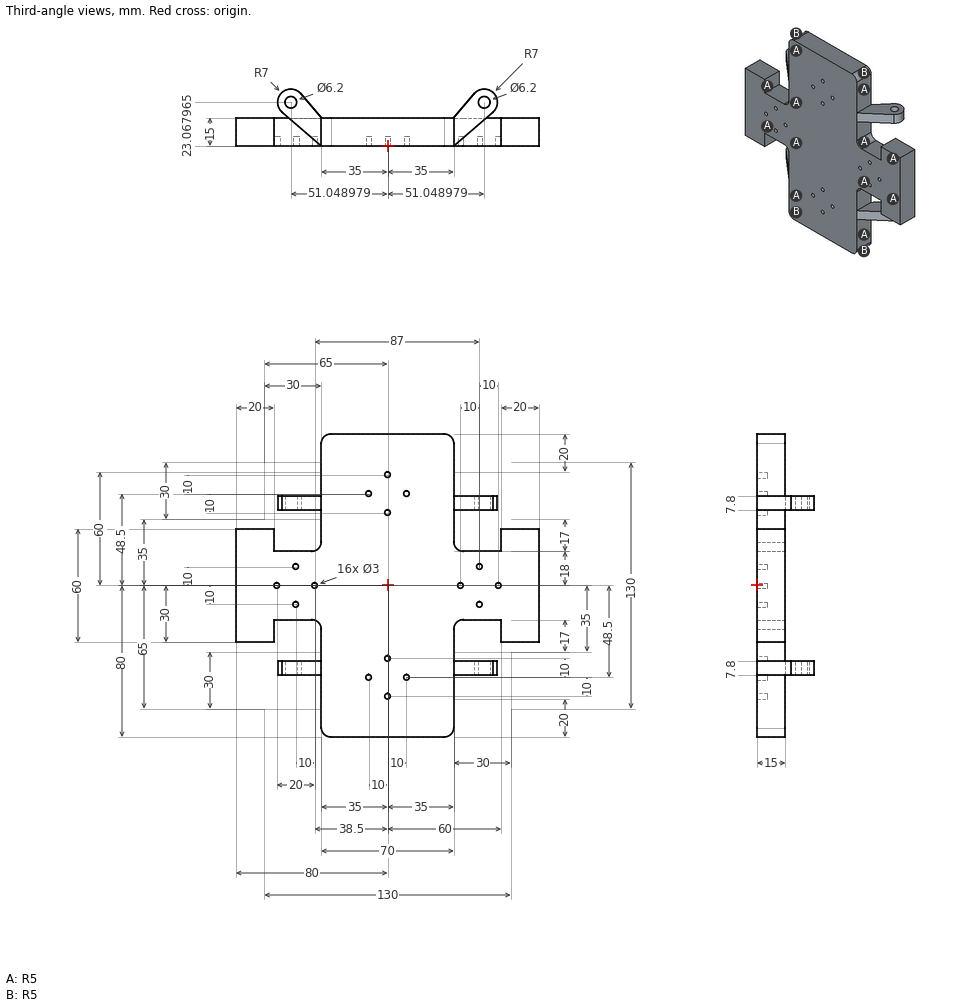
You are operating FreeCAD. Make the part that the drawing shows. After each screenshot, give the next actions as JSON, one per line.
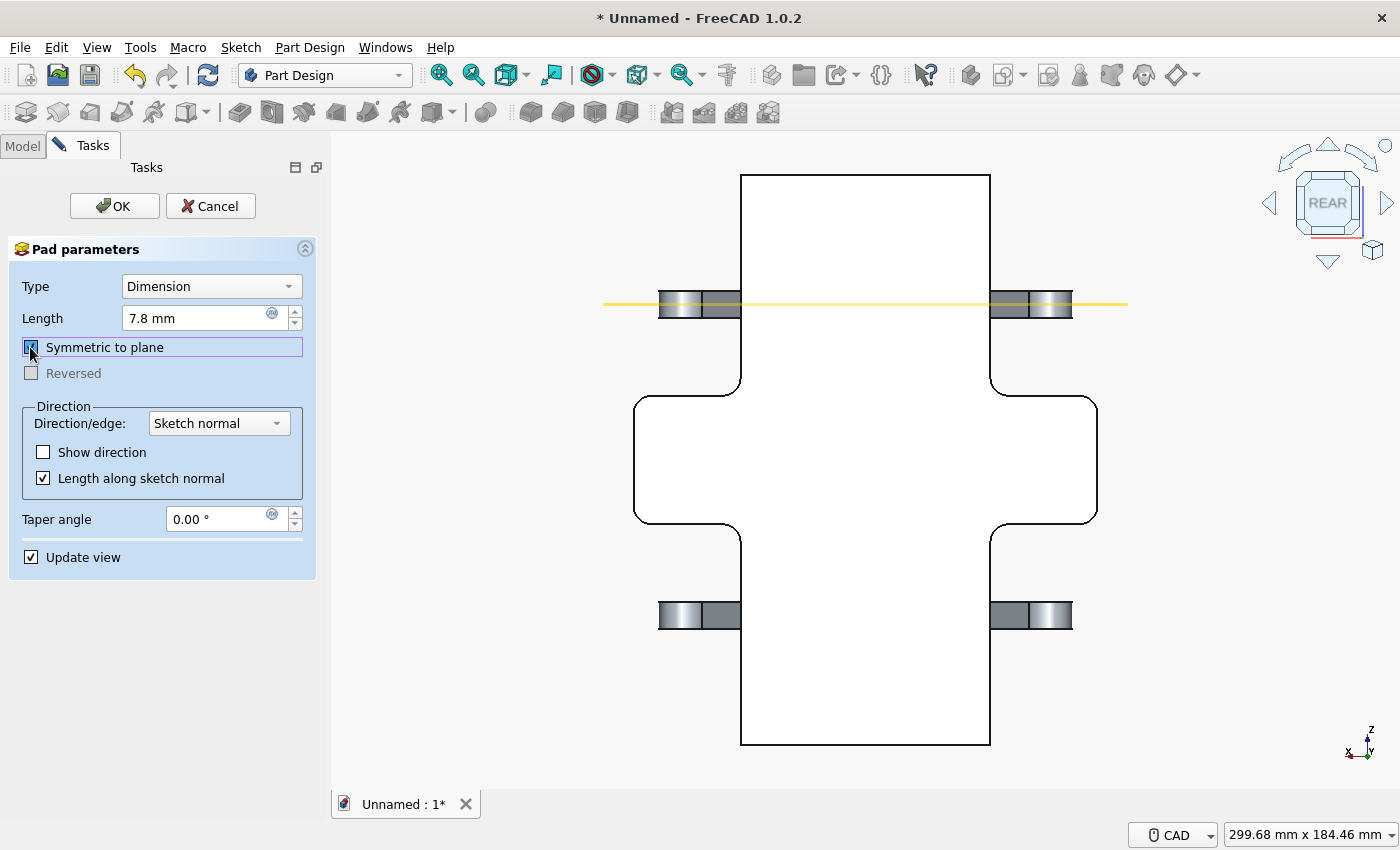
{"action": "left_click", "coordinate": [115, 206]}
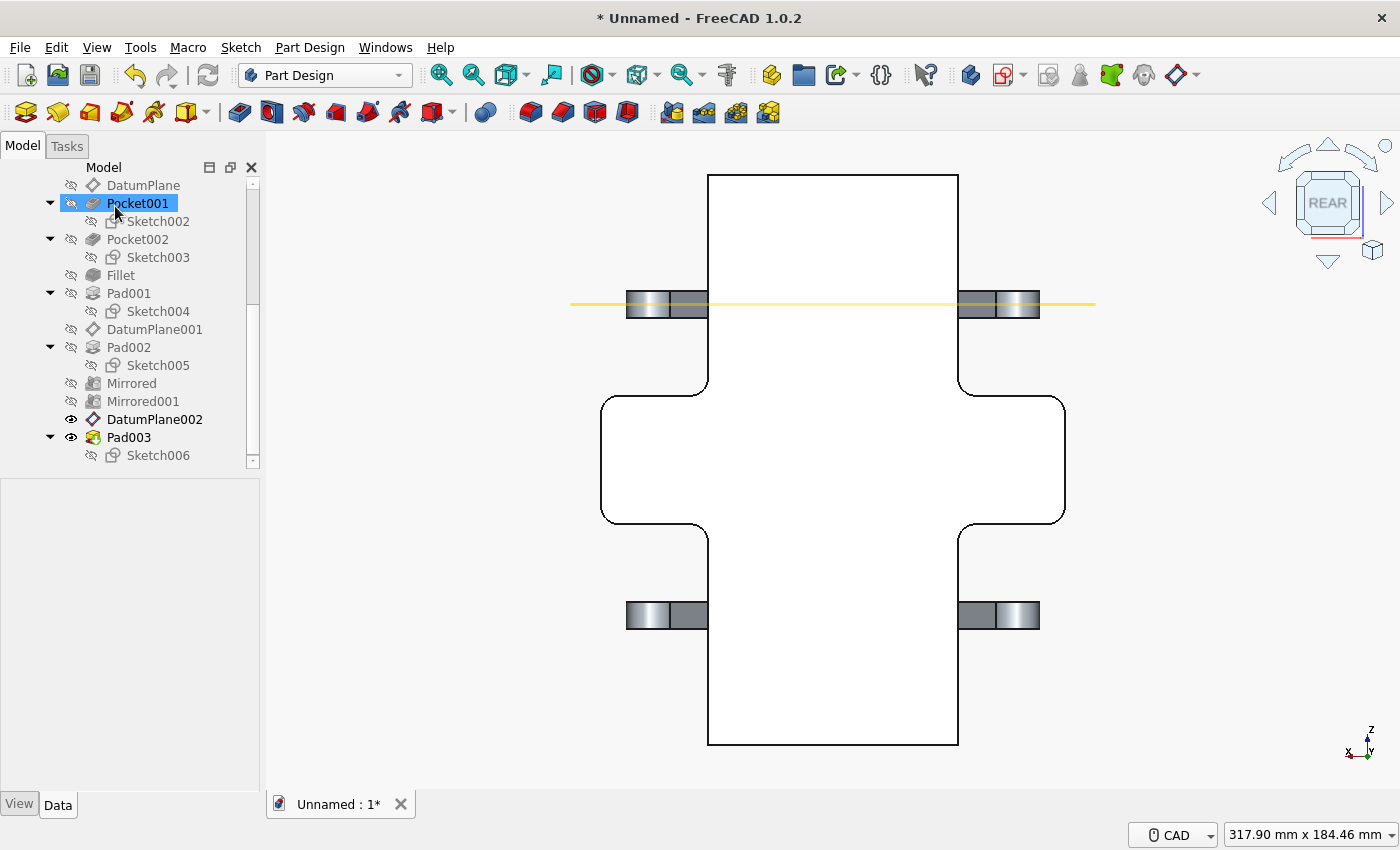
{"action": "left_click", "coordinate": [116, 419]}
{"action": "key", "text": "space"}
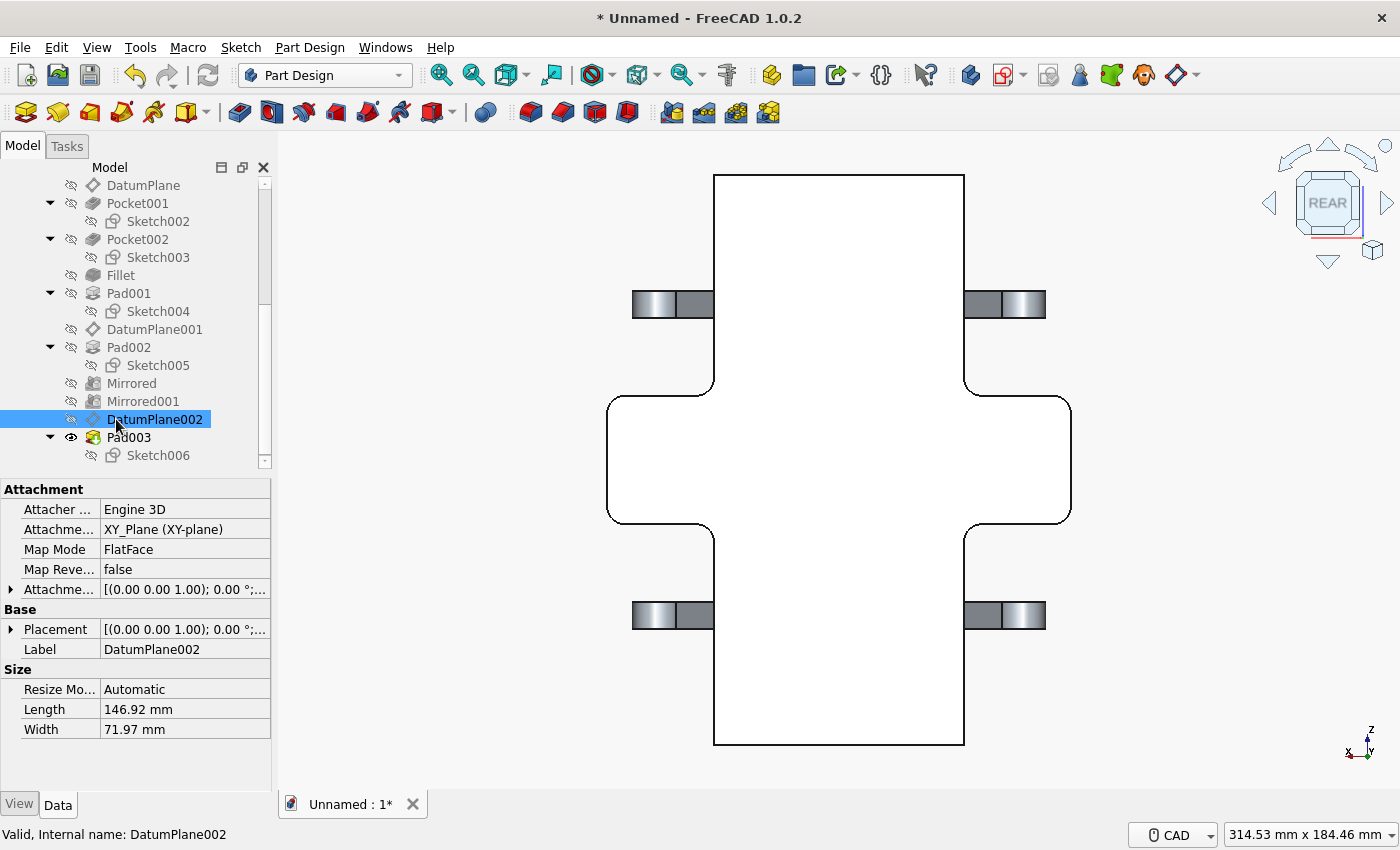
{"action": "key", "text": "0"}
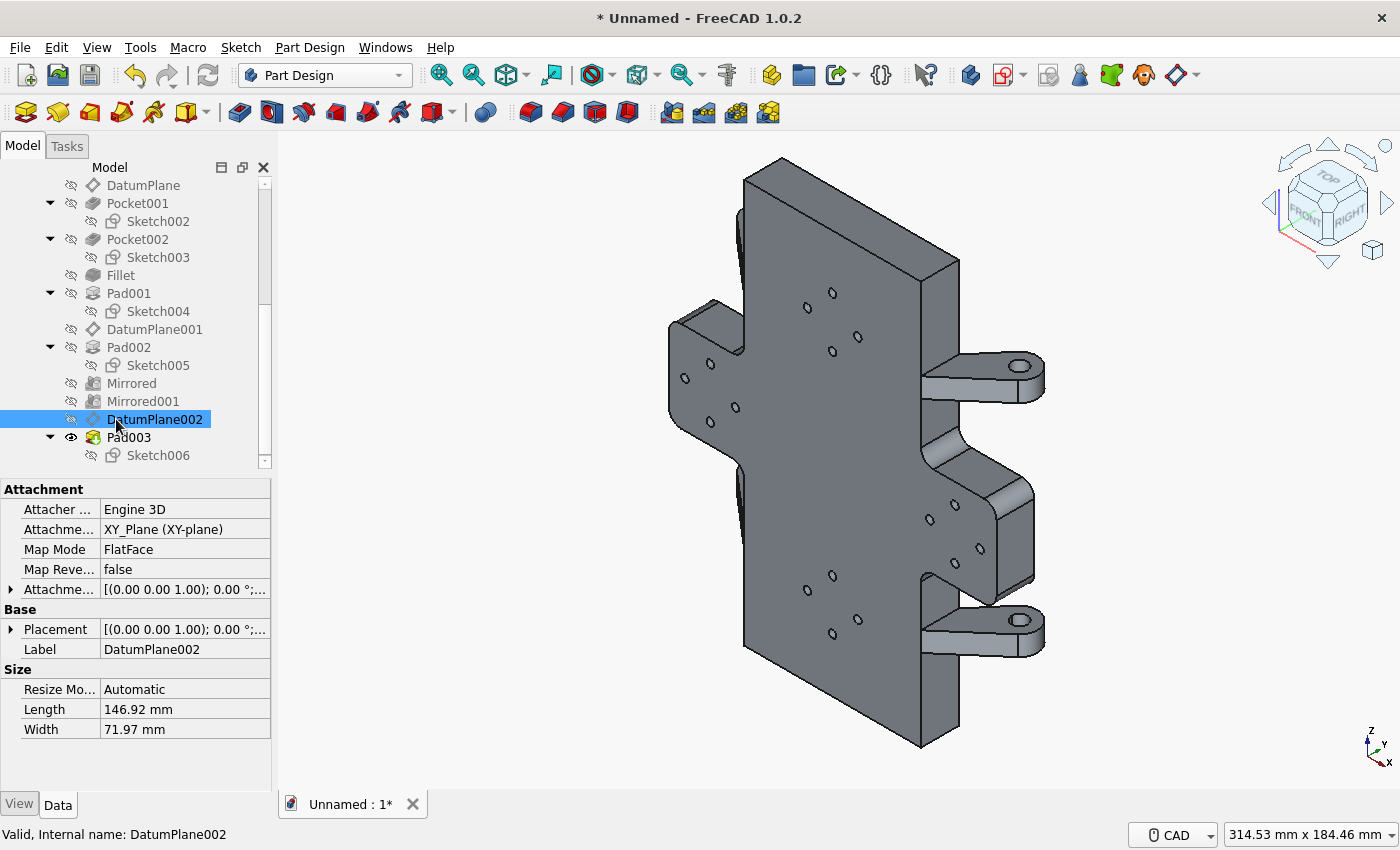
{"action": "key", "text": "v f"}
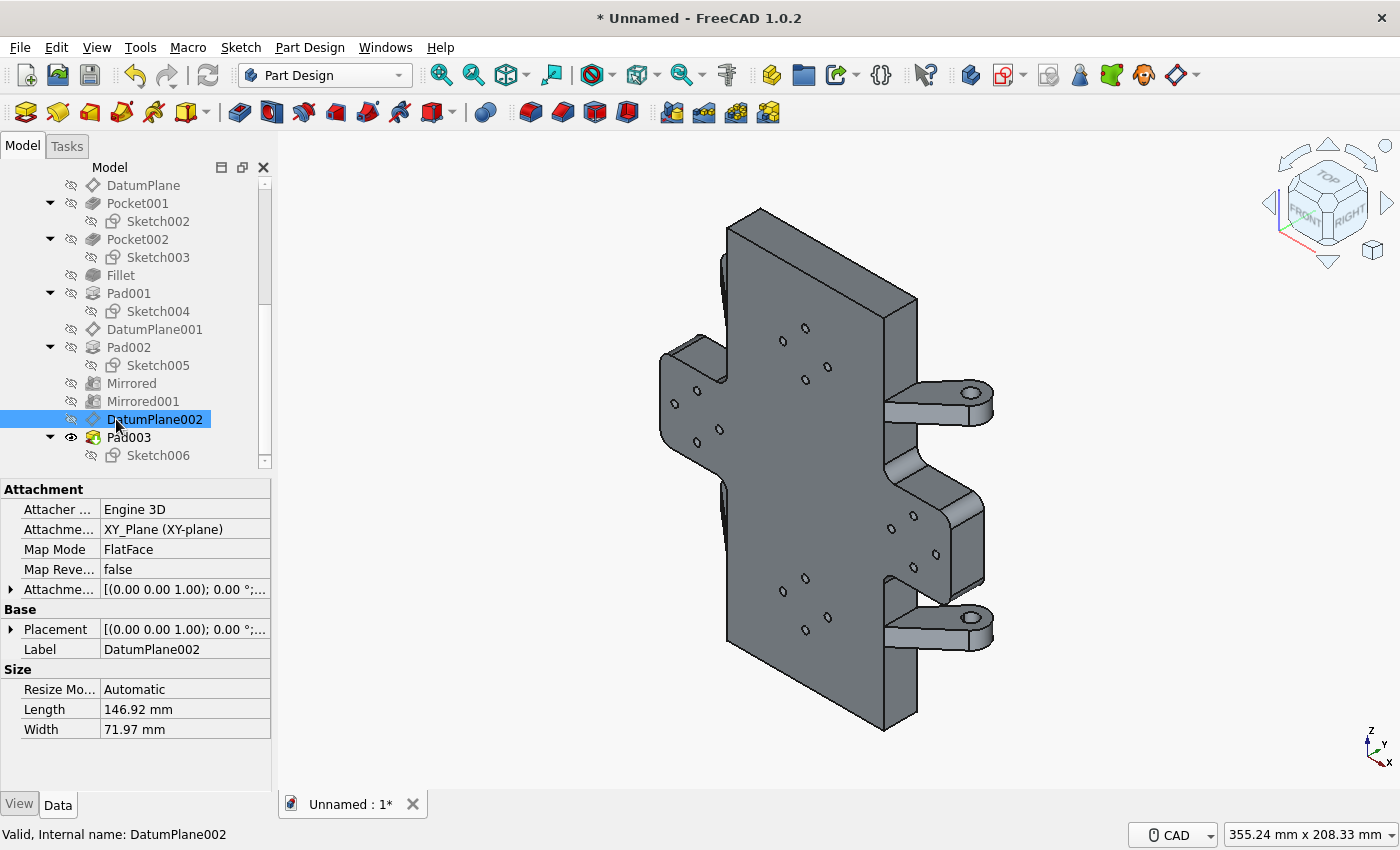
{"action": "left_click", "coordinate": [900, 308]}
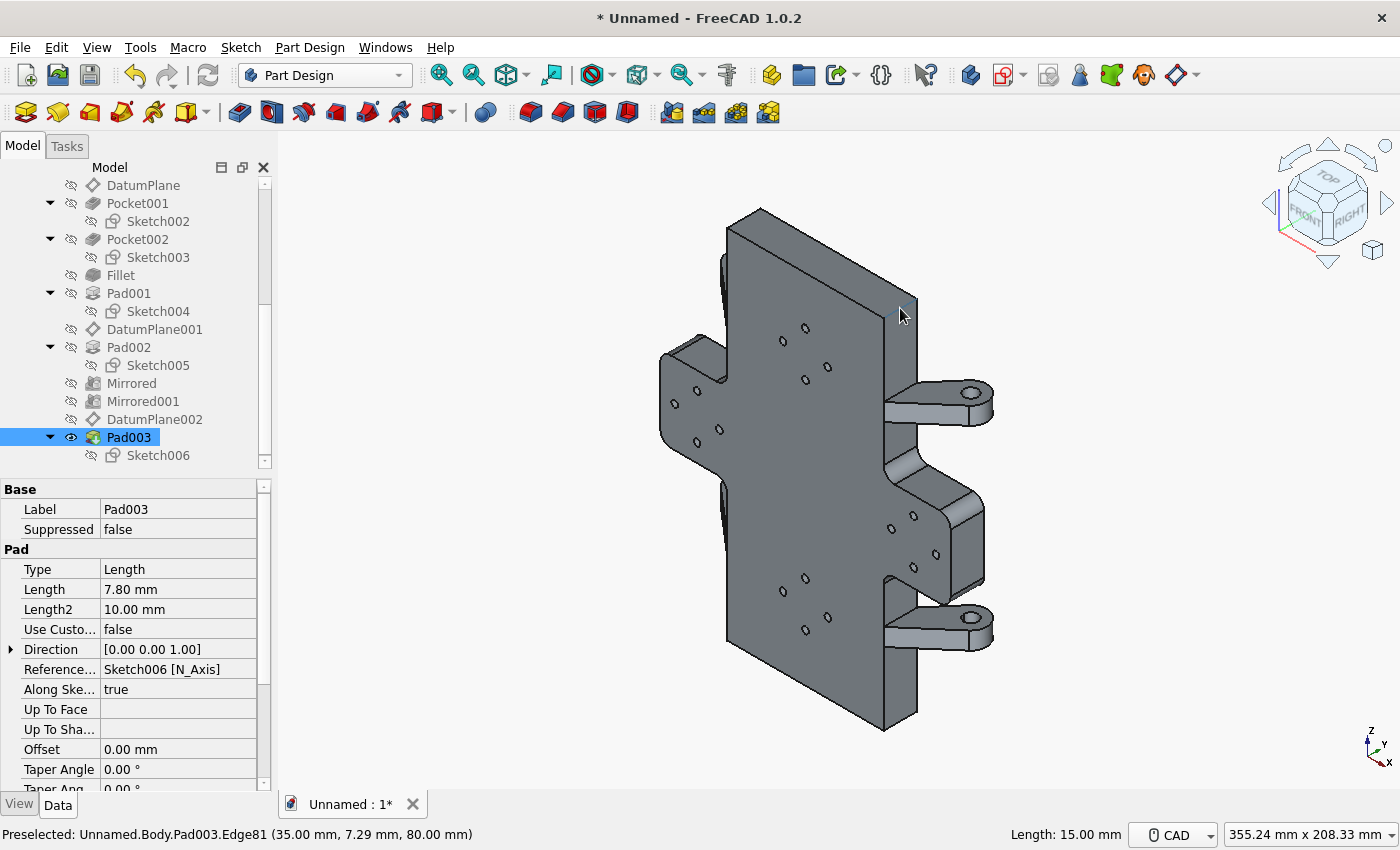
{"action": "key", "text": "2"}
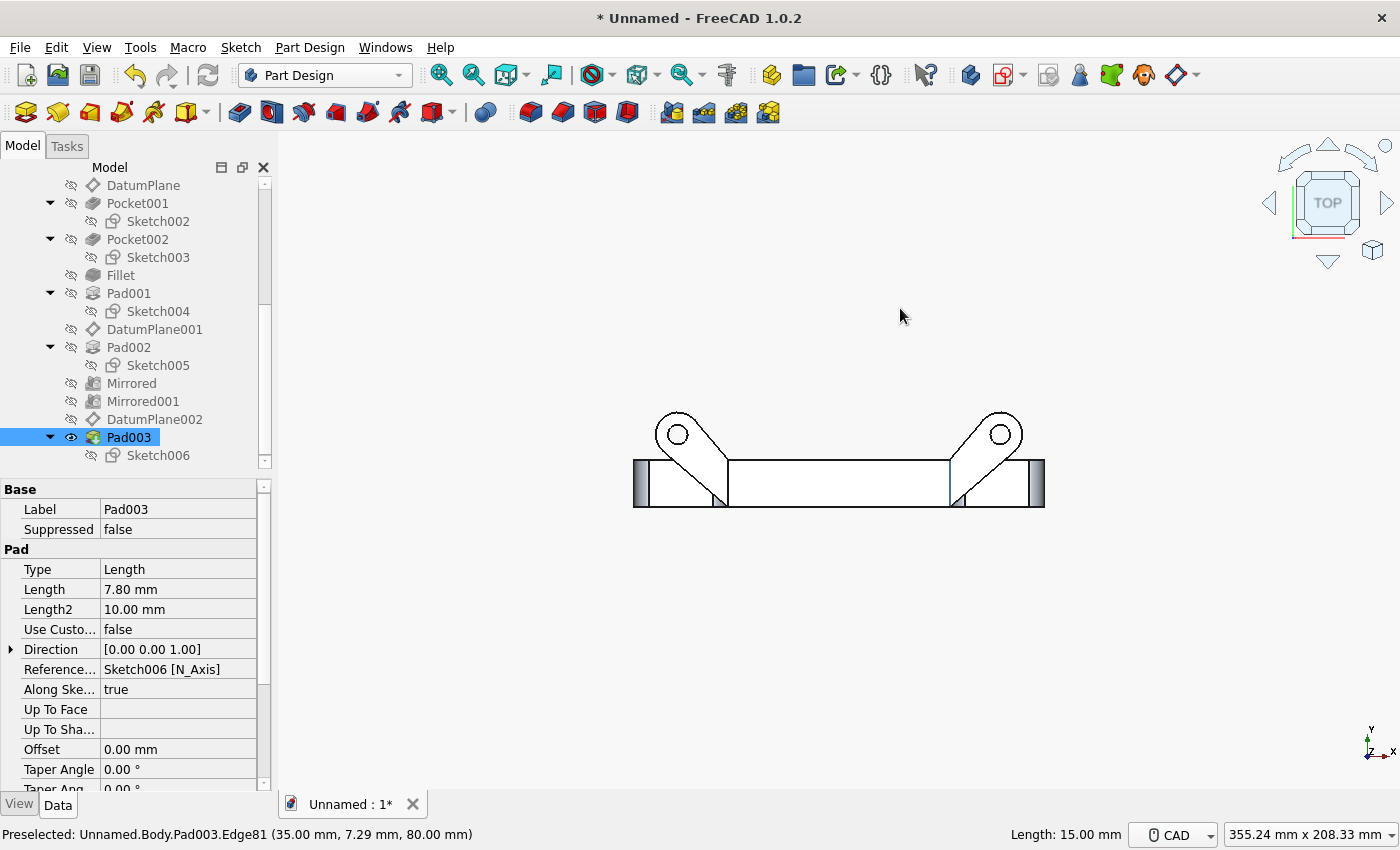
{"action": "key", "text": "v f"}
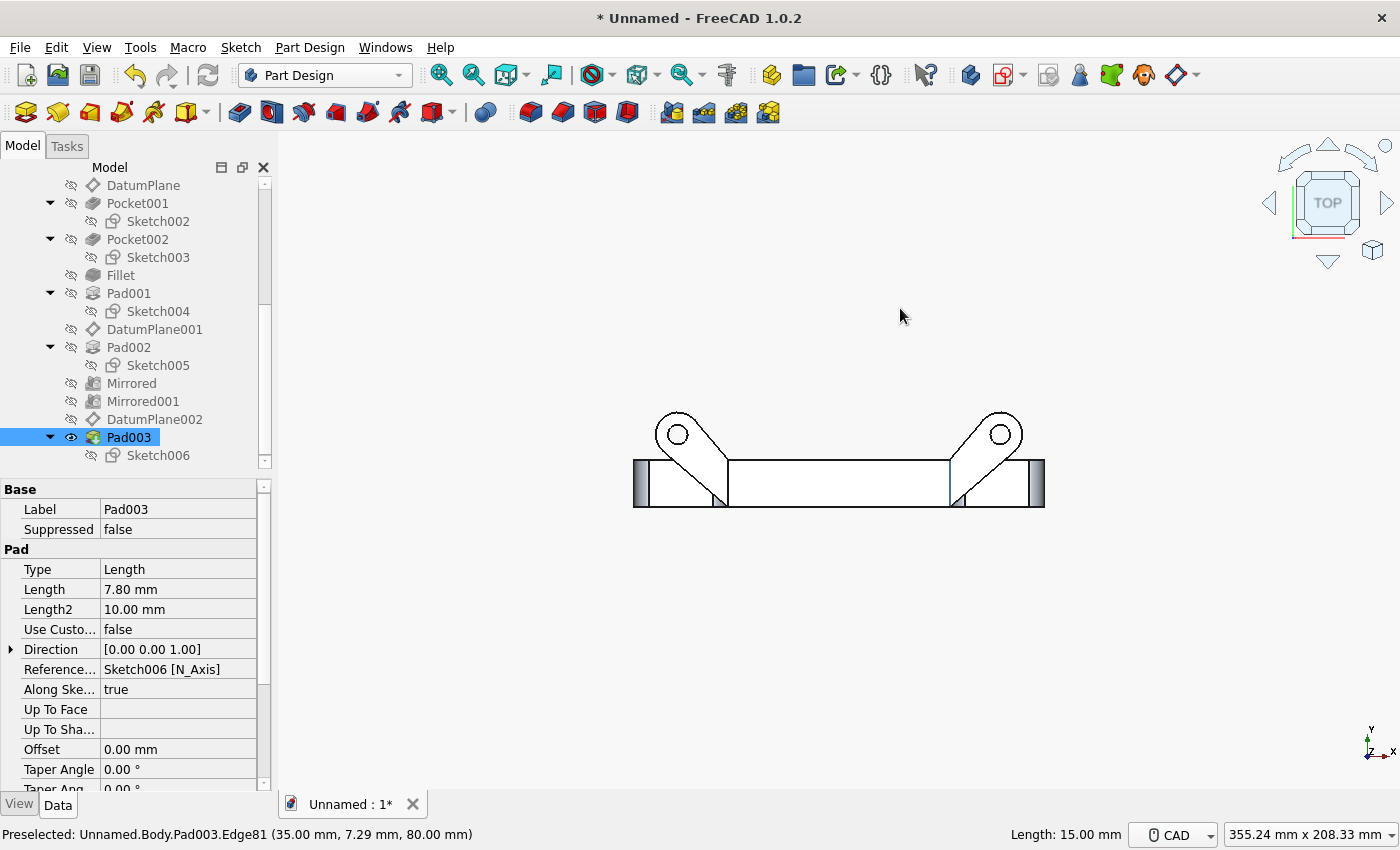
{"action": "left_click", "coordinate": [728, 483], "text": "ctrl"}